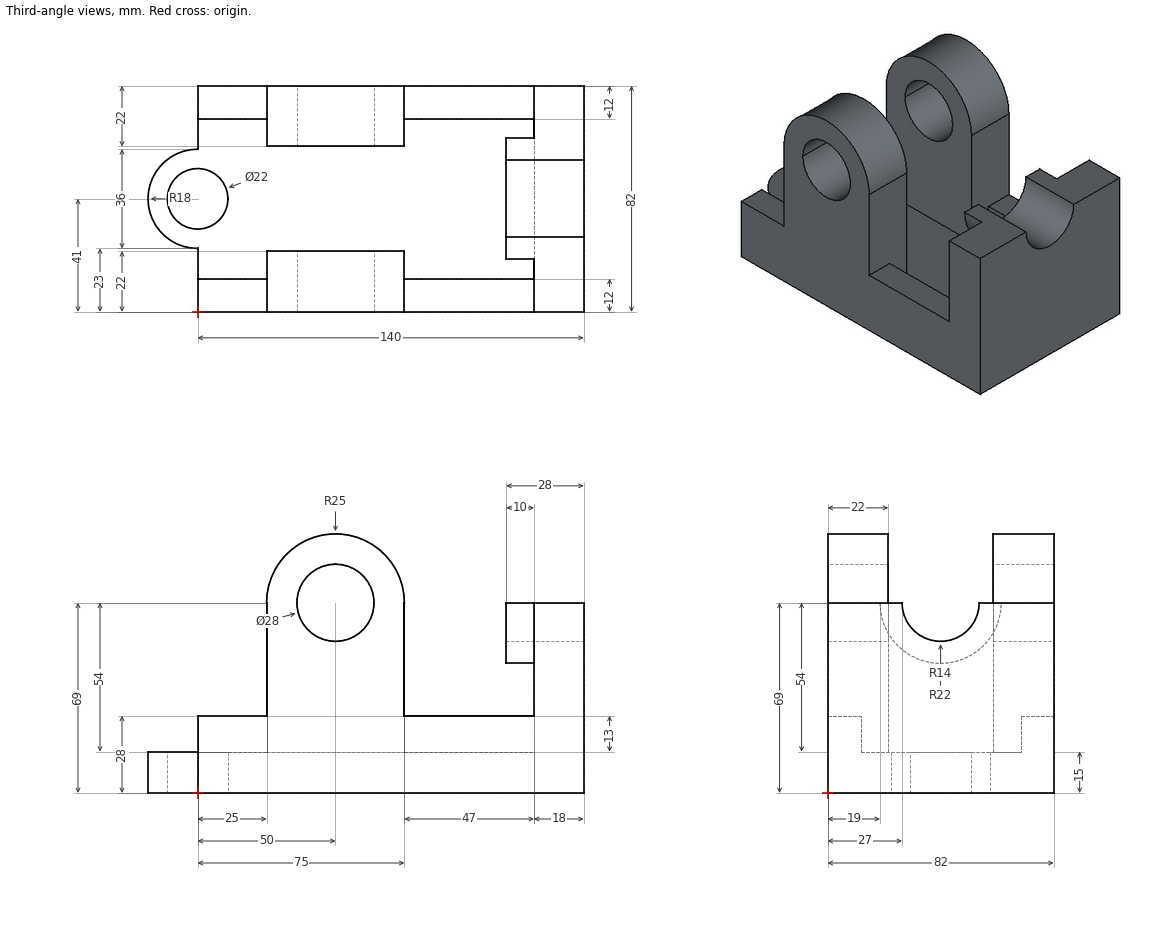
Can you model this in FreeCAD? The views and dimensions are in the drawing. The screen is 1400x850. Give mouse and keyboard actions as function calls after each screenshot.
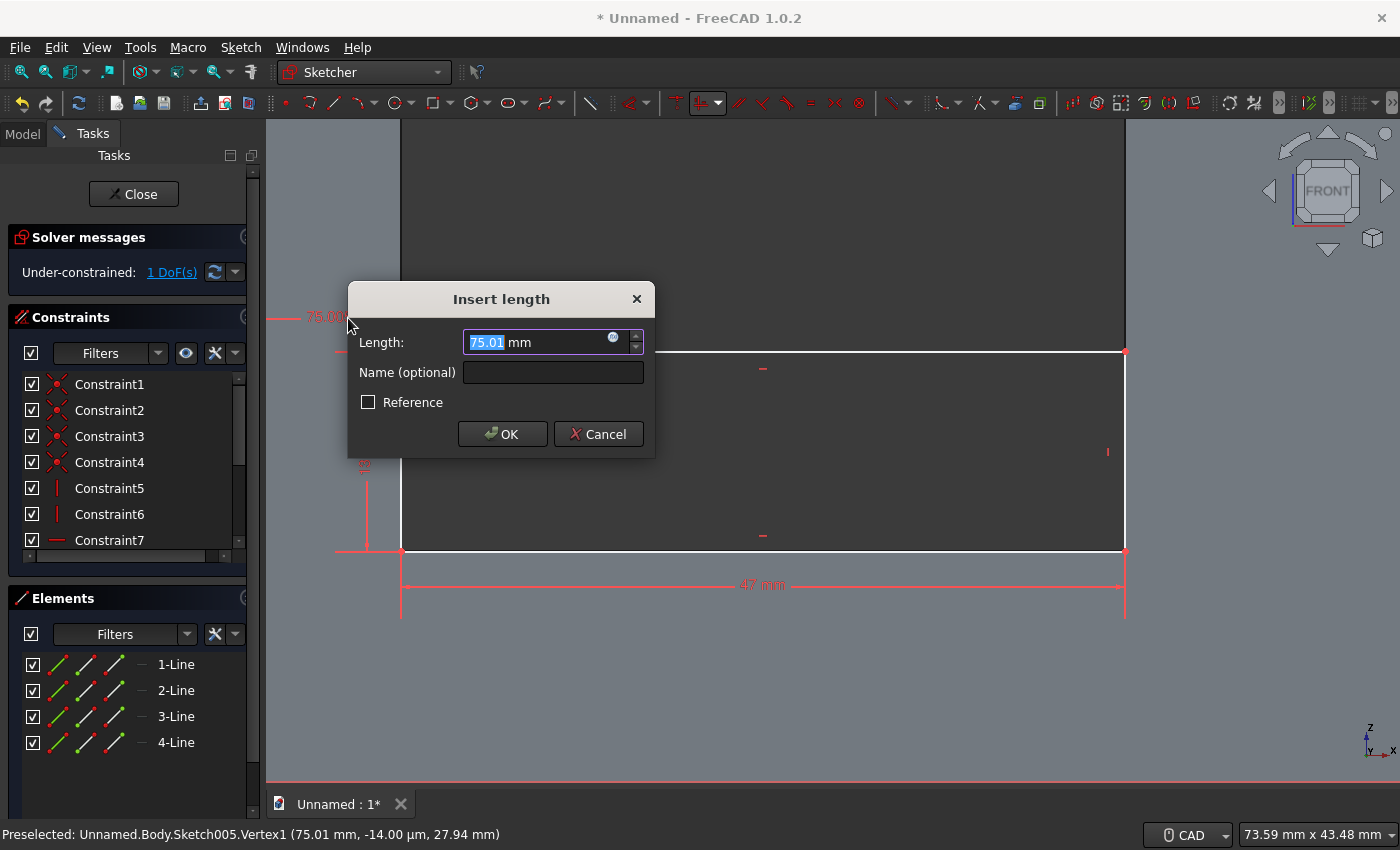
text(75)
key(Return)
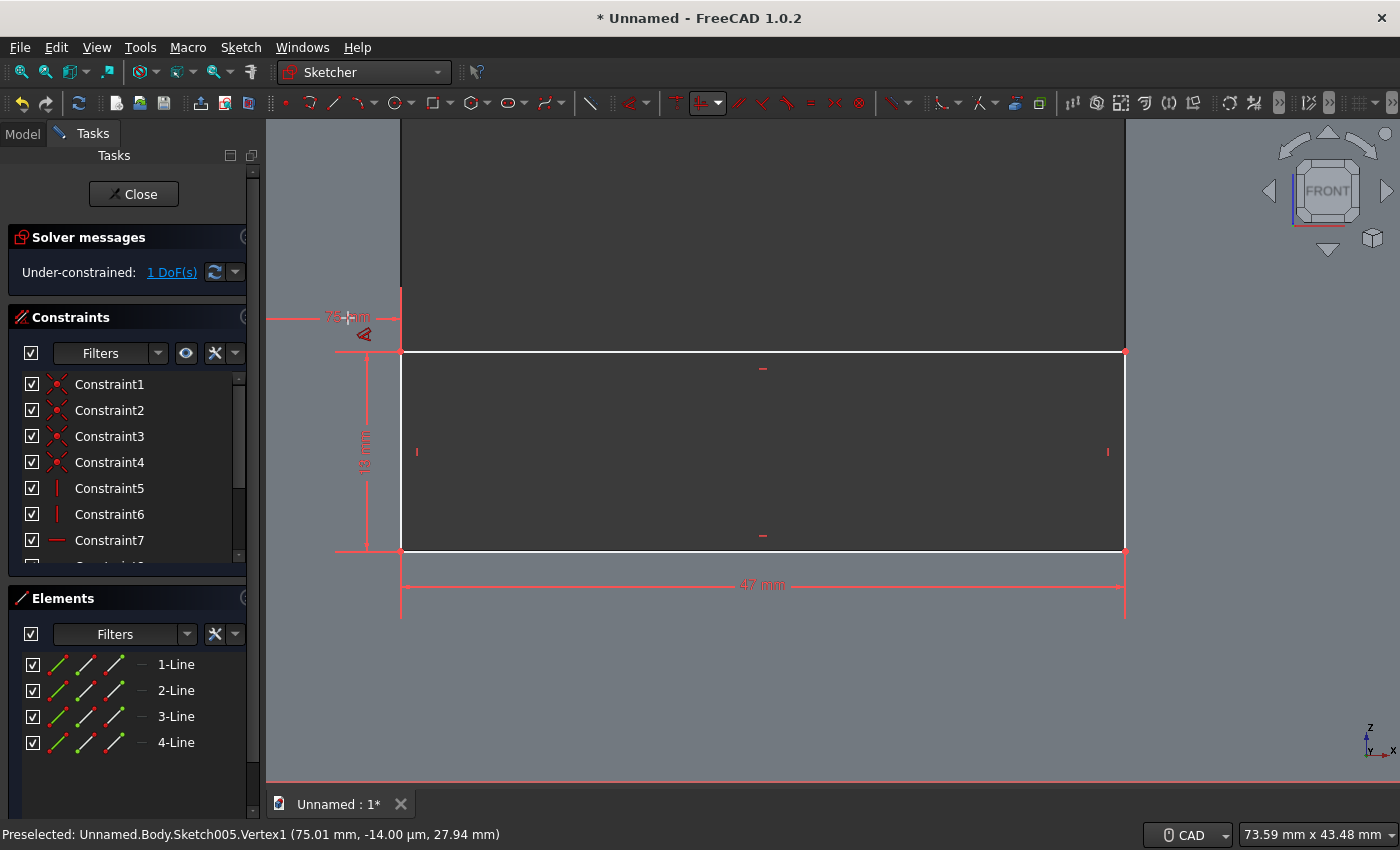
click(401, 352)
click(435, 650)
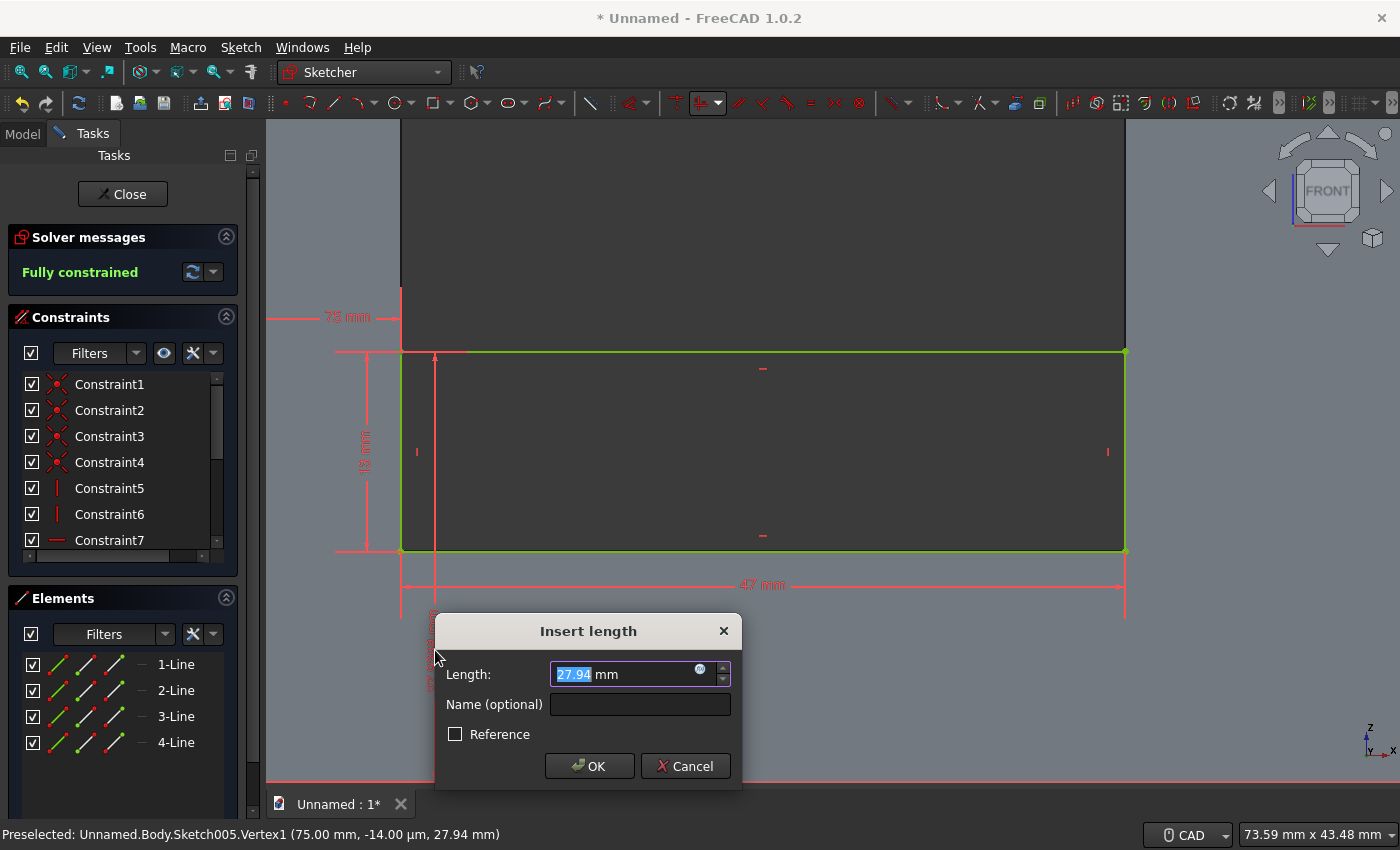
text(28)
key(Return)
key(Escape)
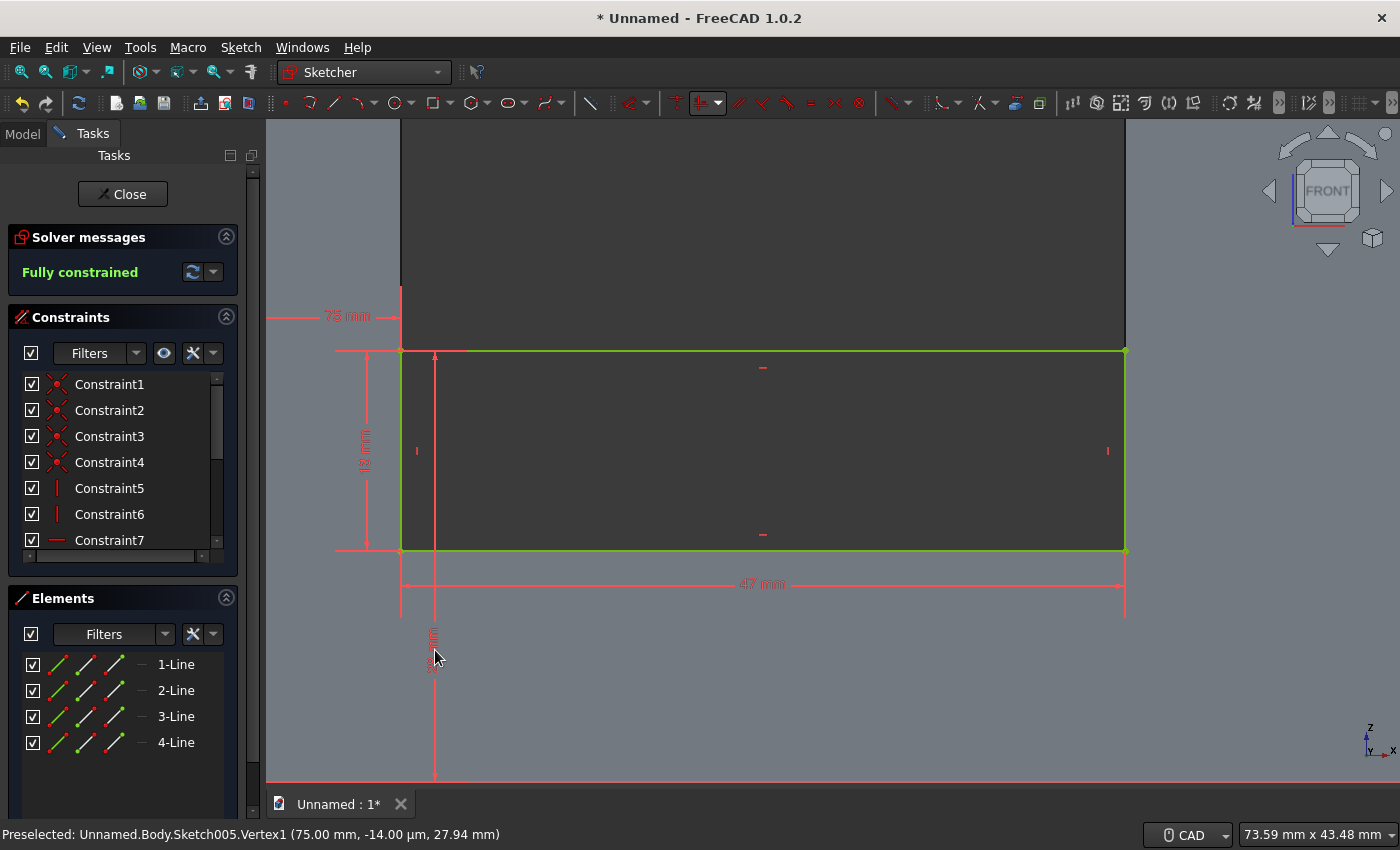
click(123, 194)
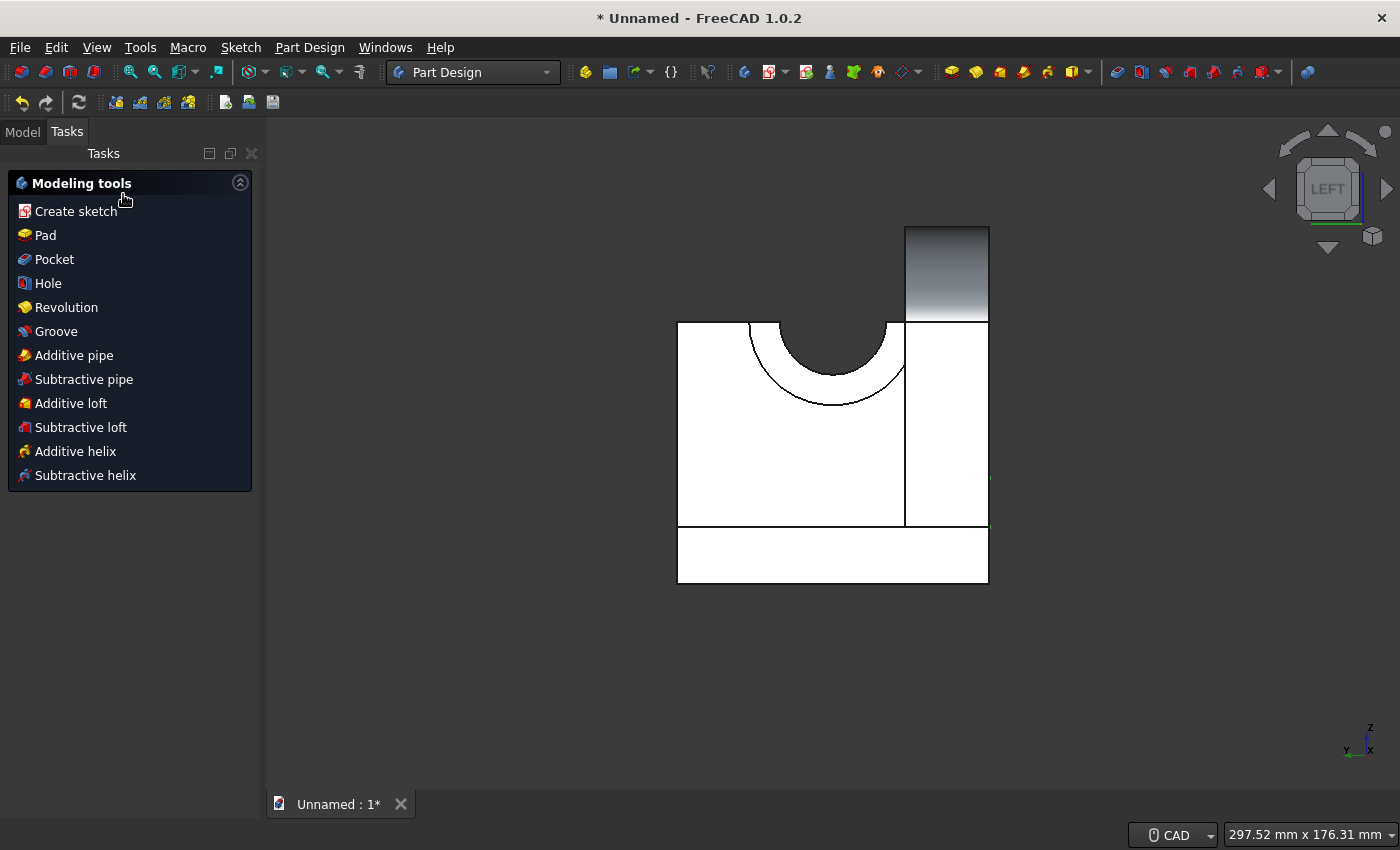
click(952, 72)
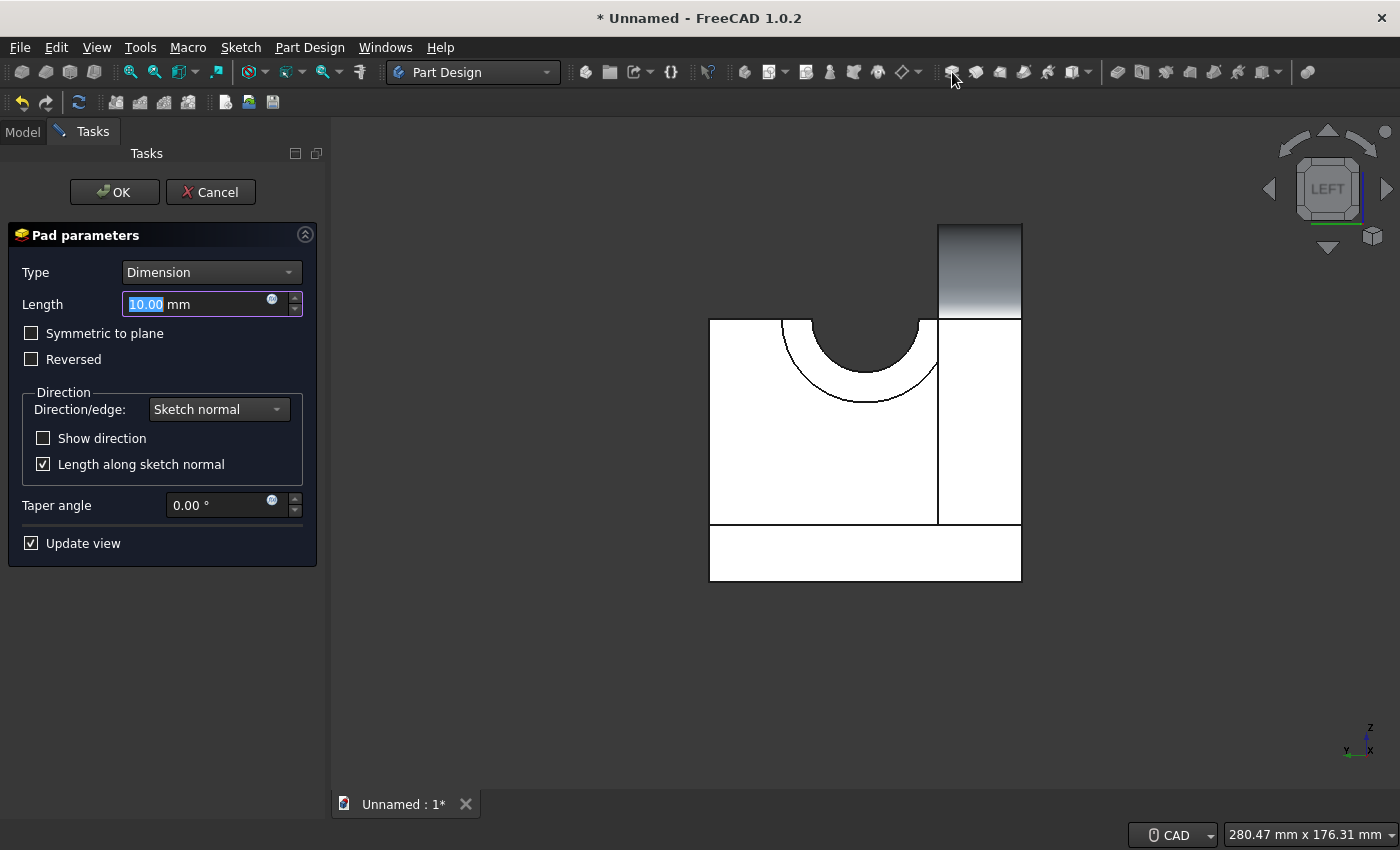
text(12)
key(Tab)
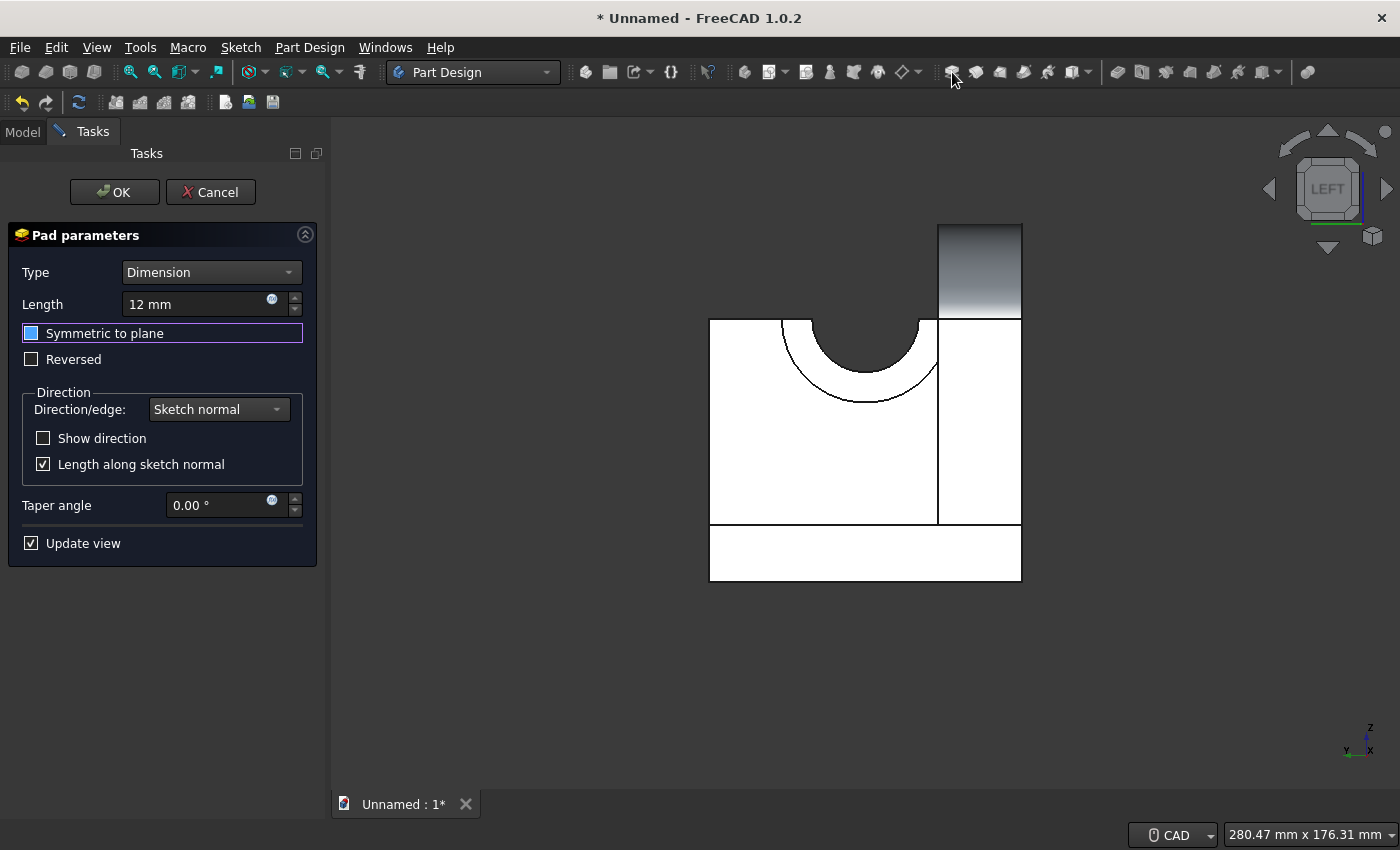
click(30, 359)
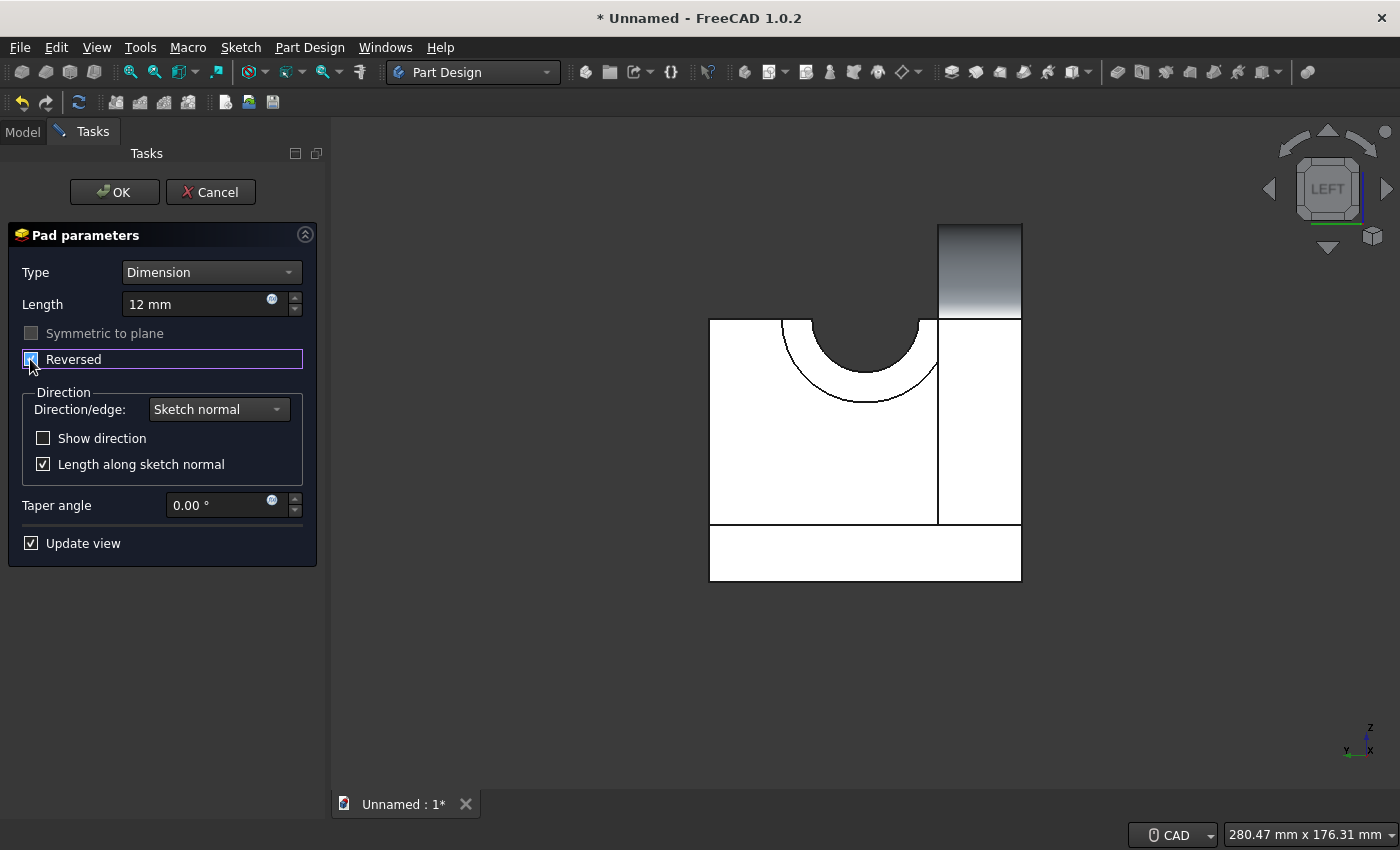
click(115, 192)